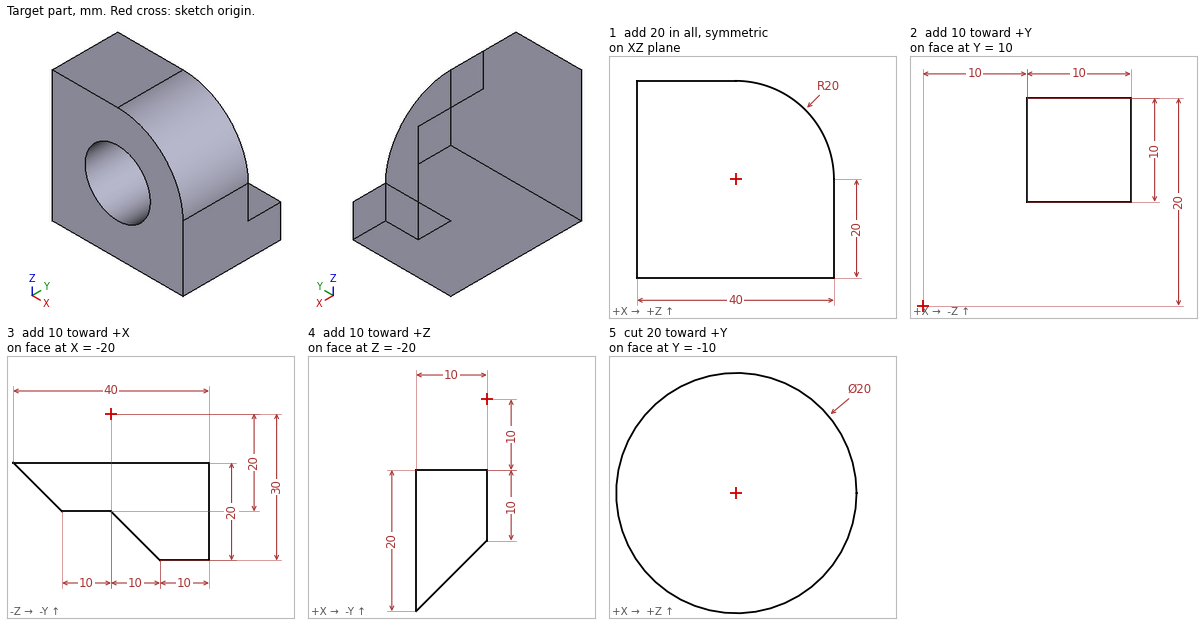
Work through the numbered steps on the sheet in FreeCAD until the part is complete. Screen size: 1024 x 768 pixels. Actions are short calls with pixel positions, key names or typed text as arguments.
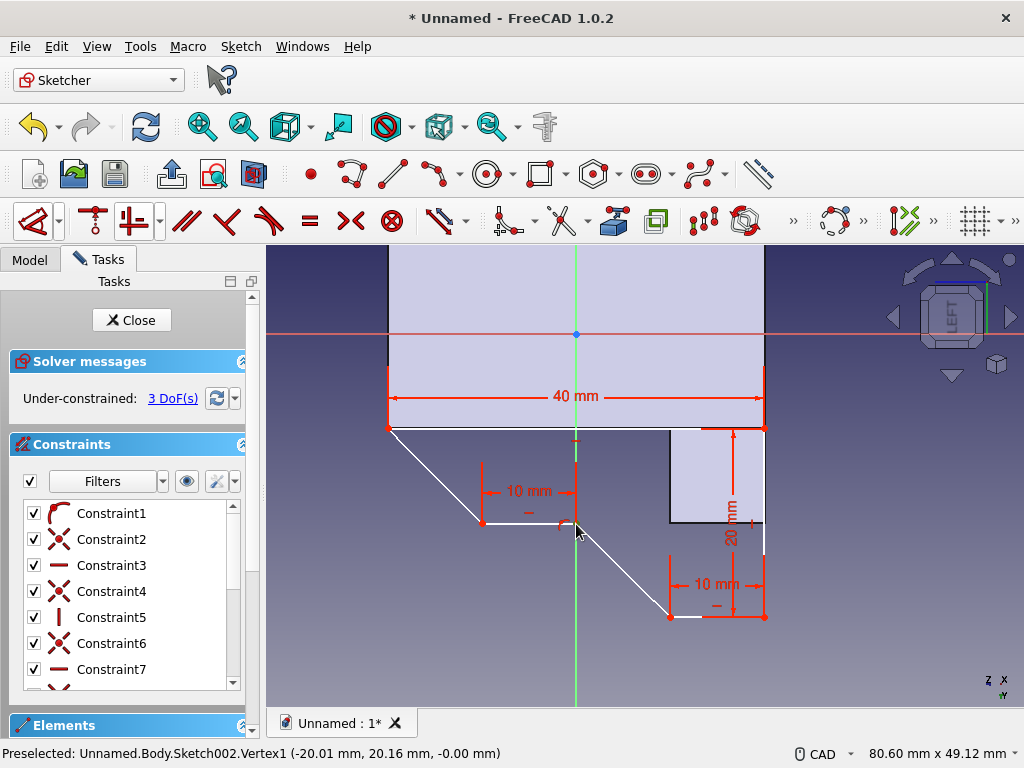
click(58, 222)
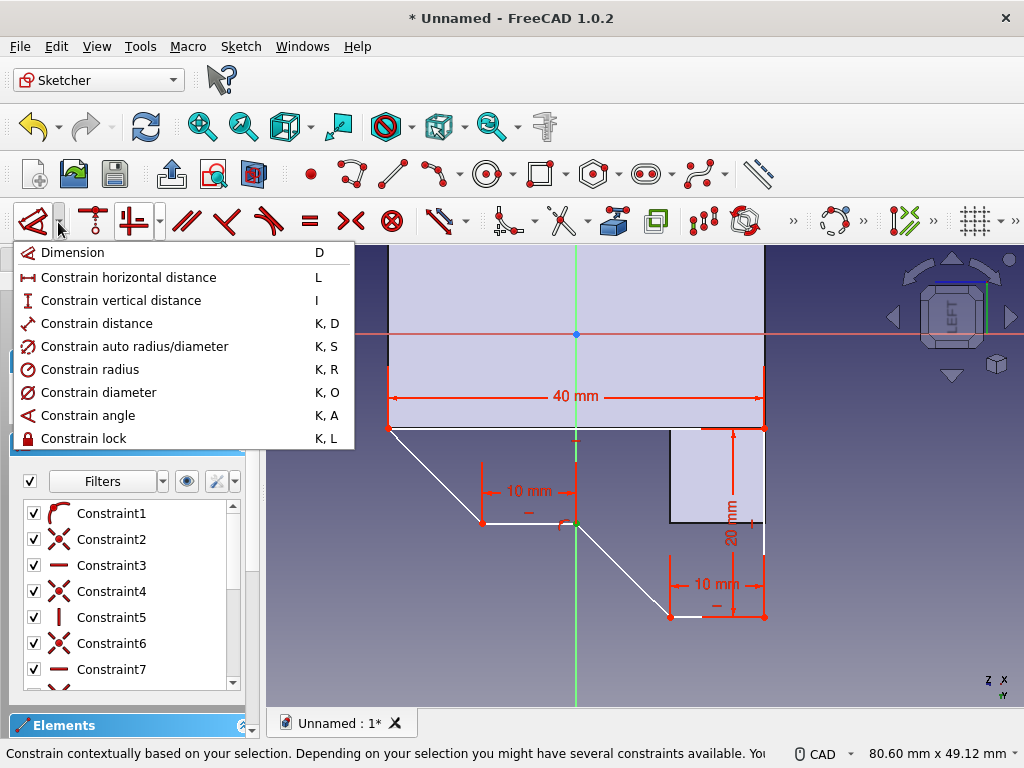
click(184, 300)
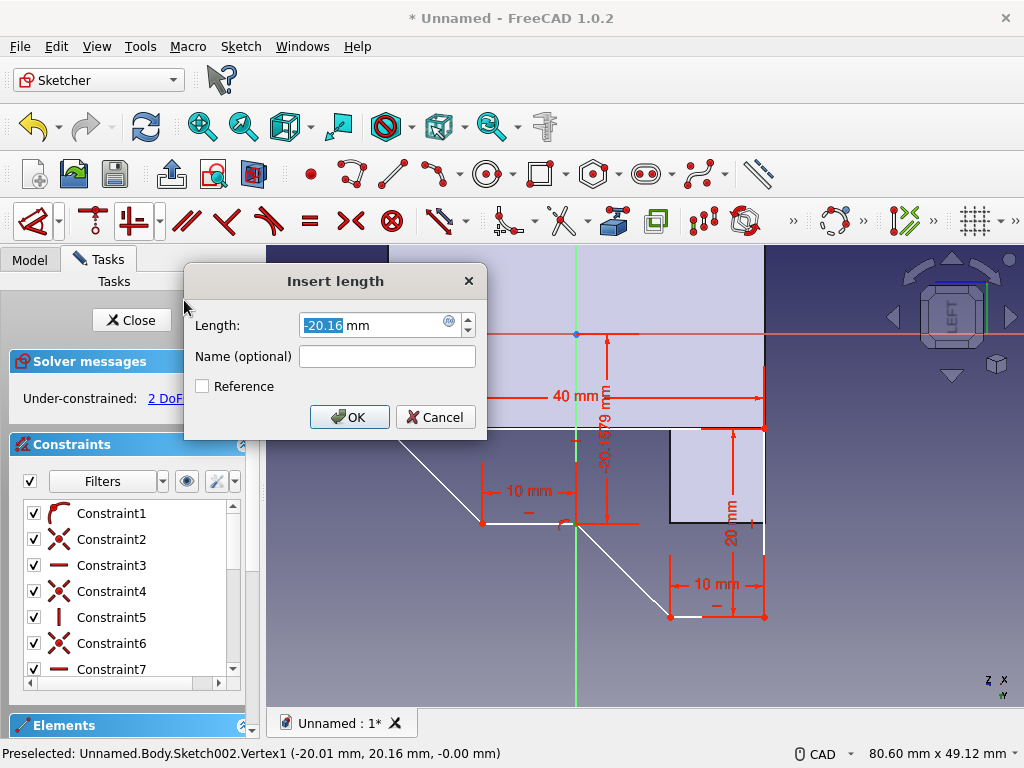
text(-20)
key(Return)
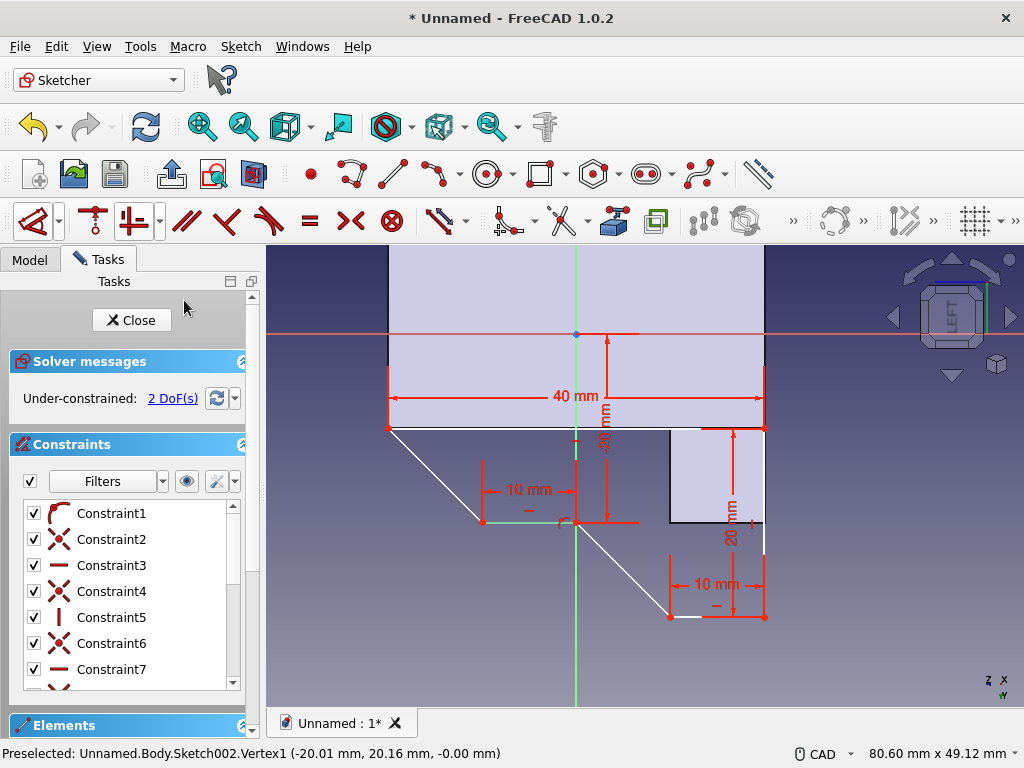
click(670, 617)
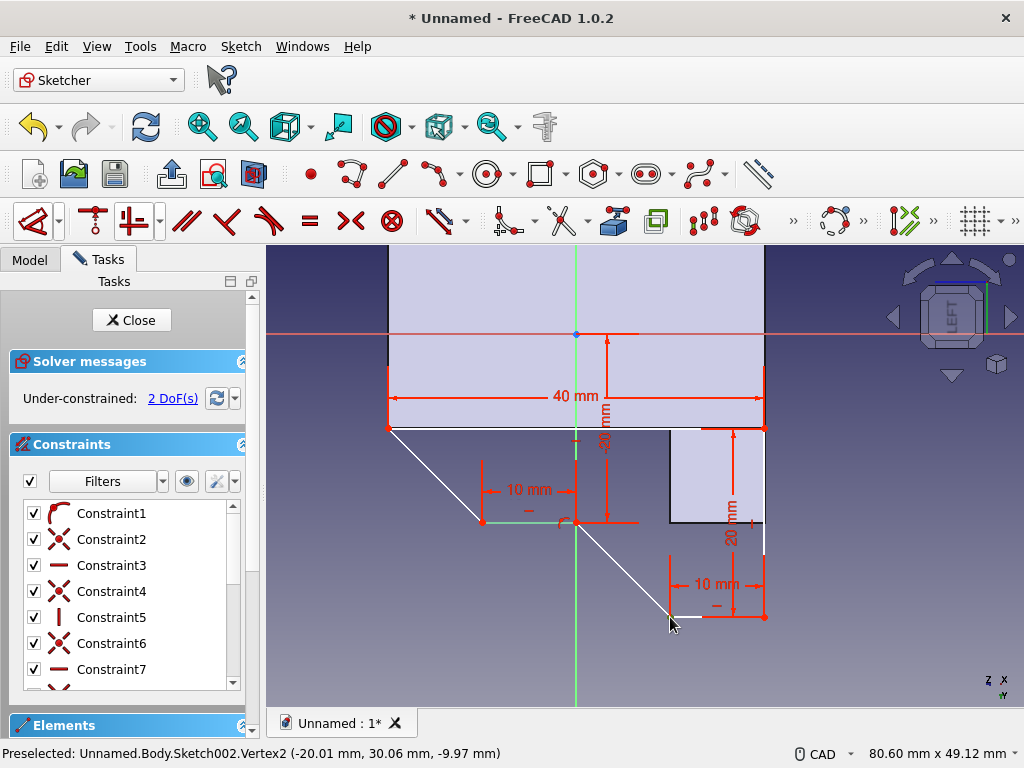
key(l)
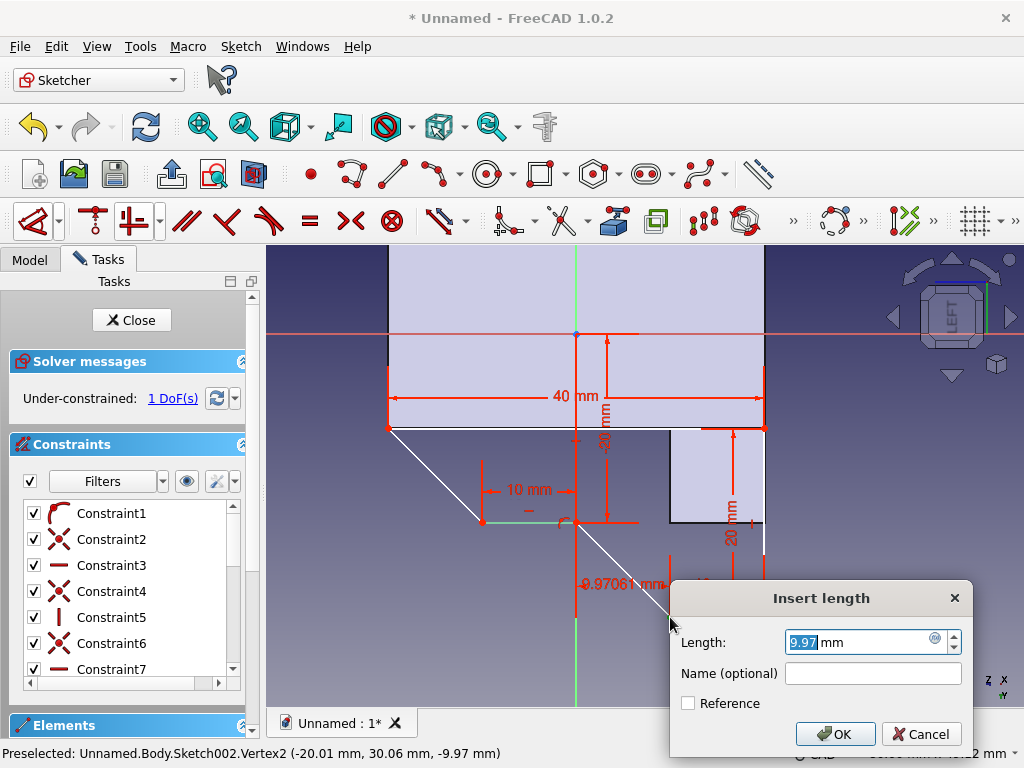
text(10)
key(Return)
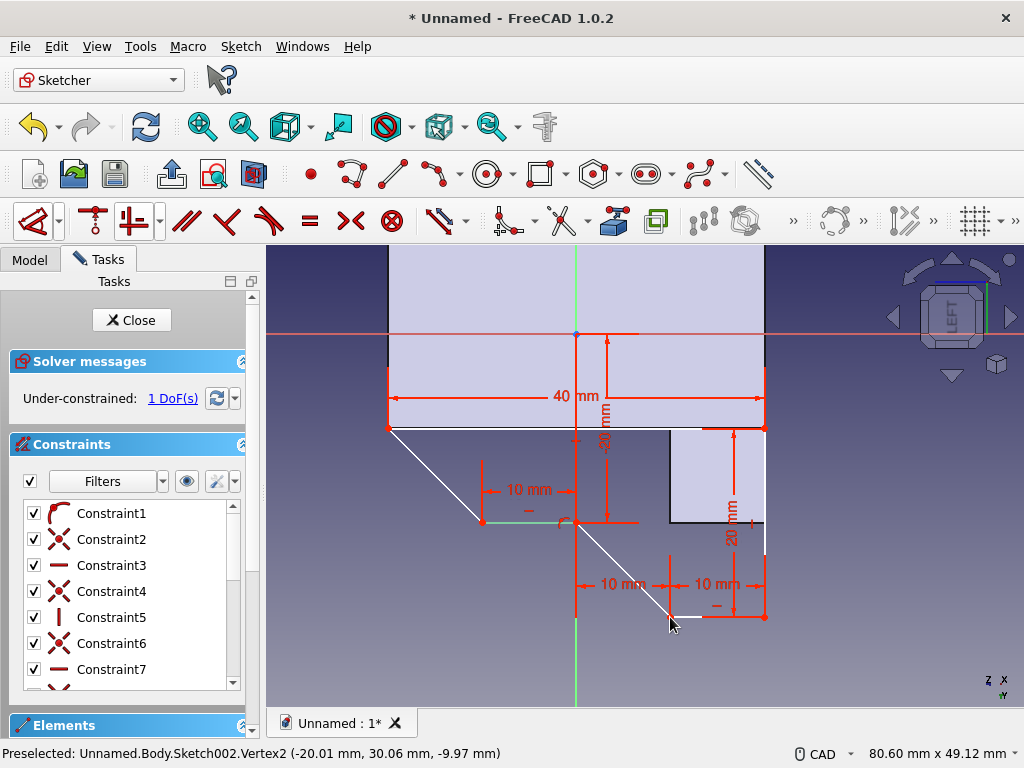
click(670, 617)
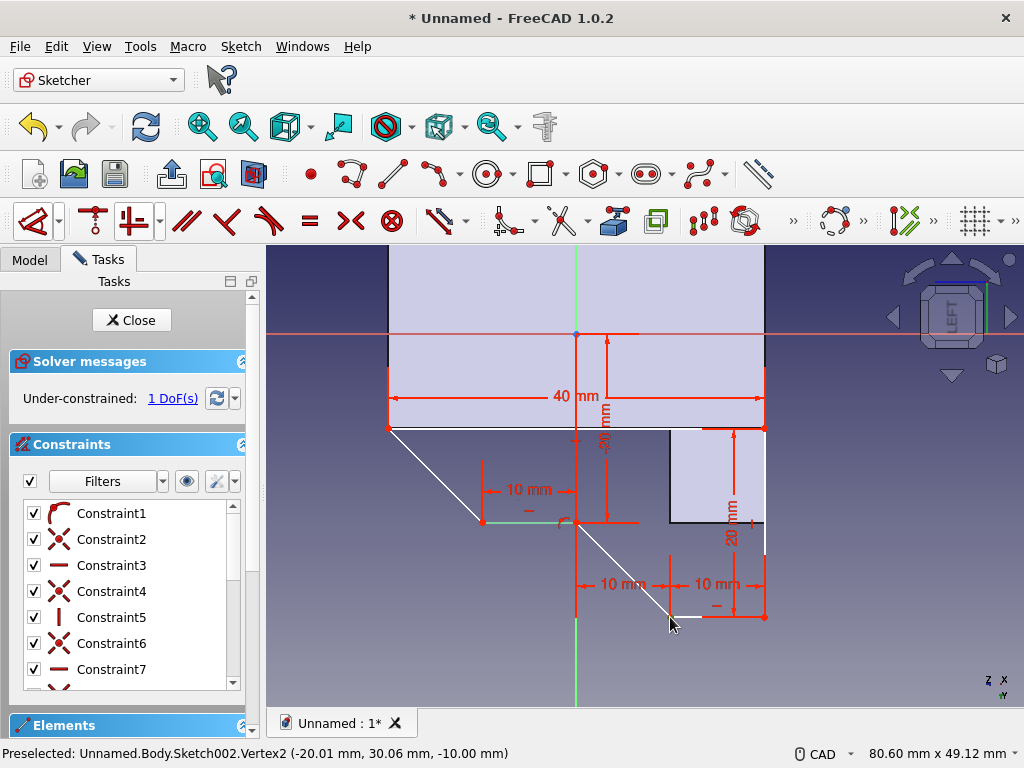
click(58, 222)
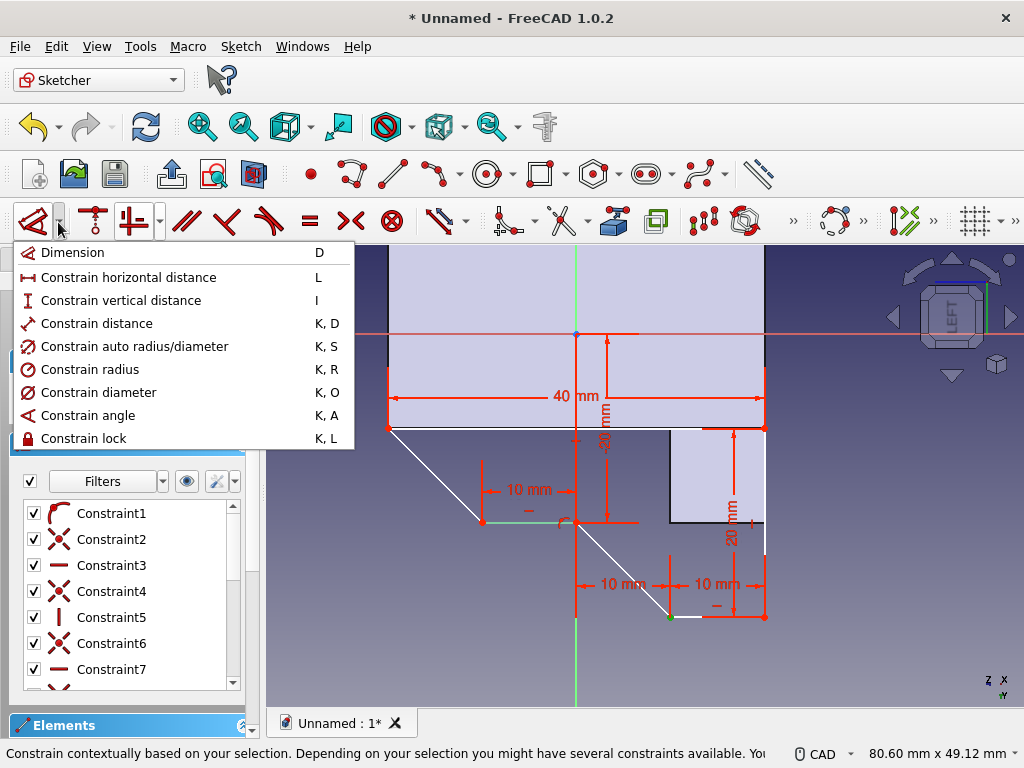
click(184, 300)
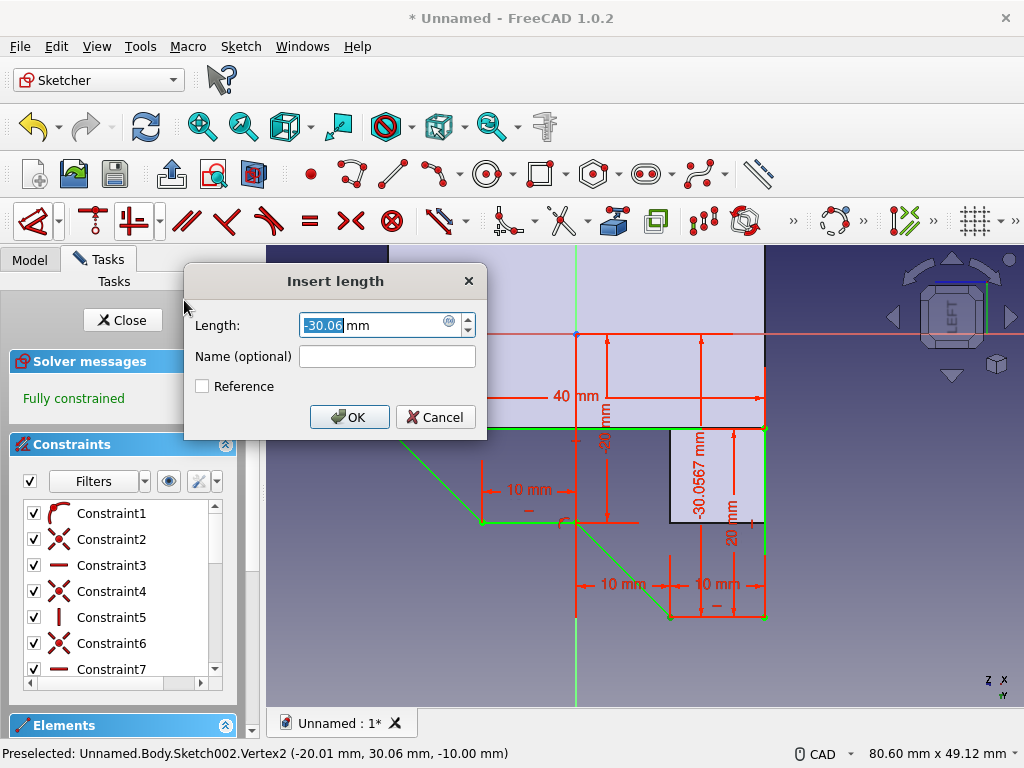
text(-30)
key(Return)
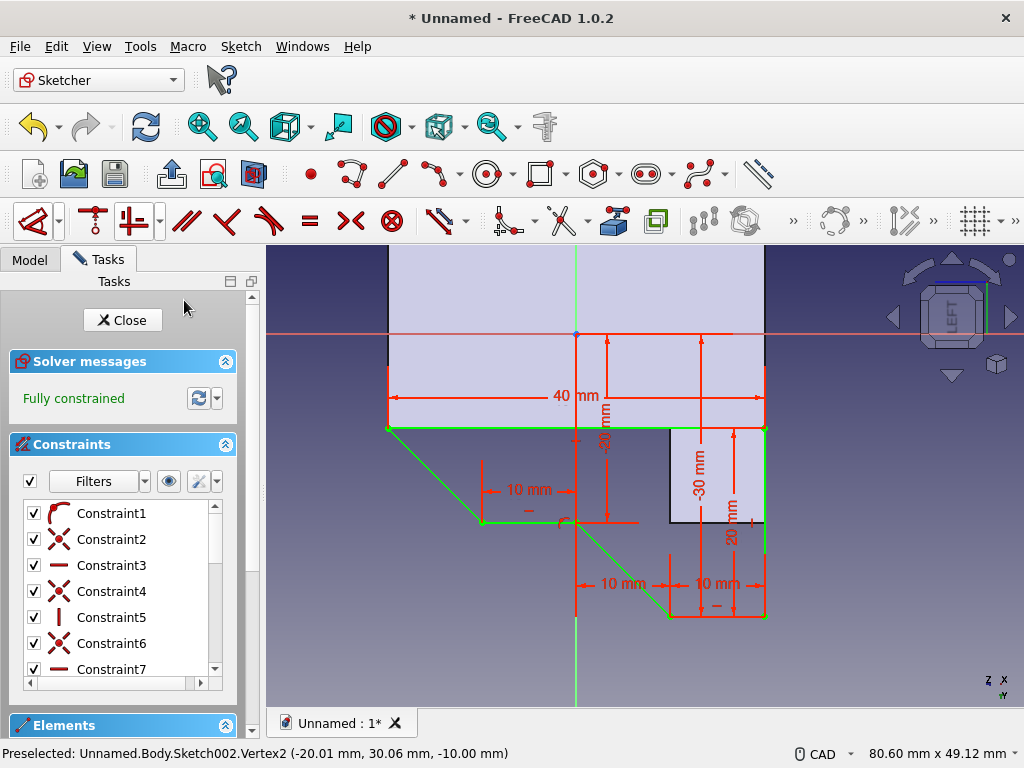
click(123, 320)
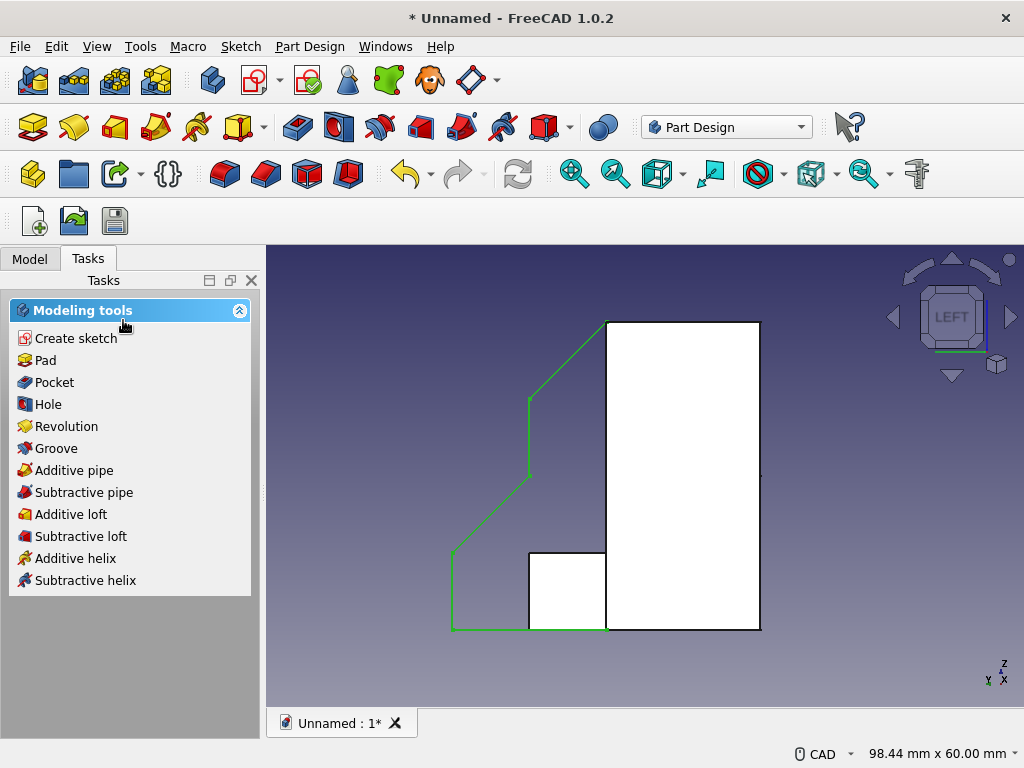
click(33, 128)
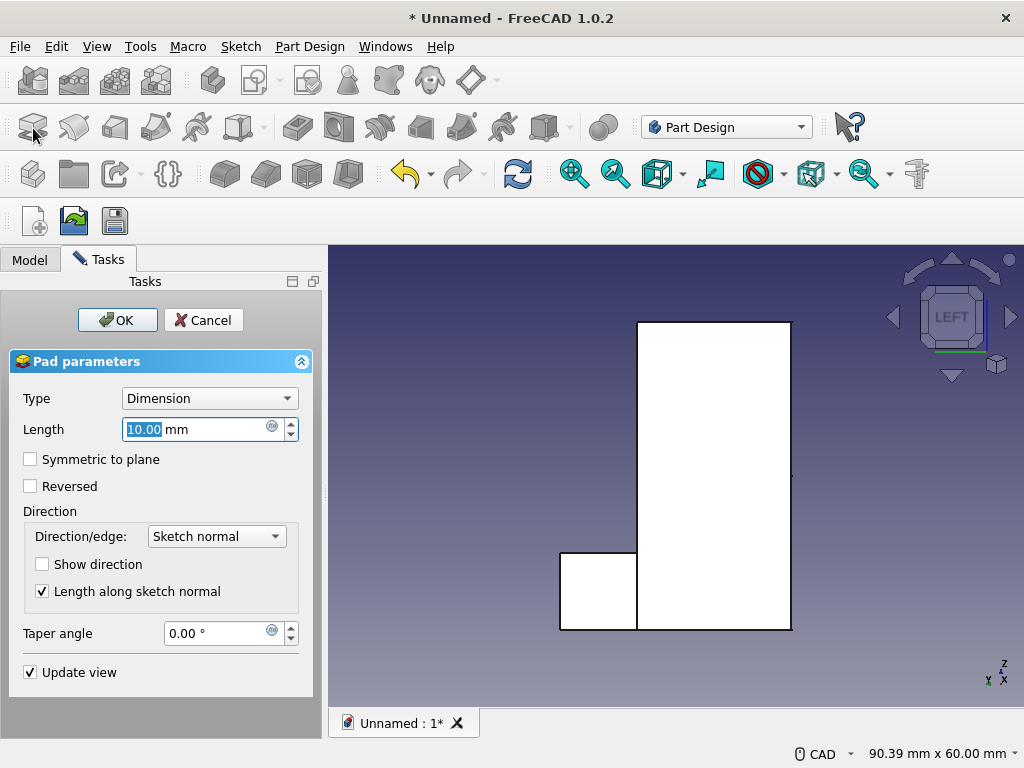
text(10)
key(Tab)